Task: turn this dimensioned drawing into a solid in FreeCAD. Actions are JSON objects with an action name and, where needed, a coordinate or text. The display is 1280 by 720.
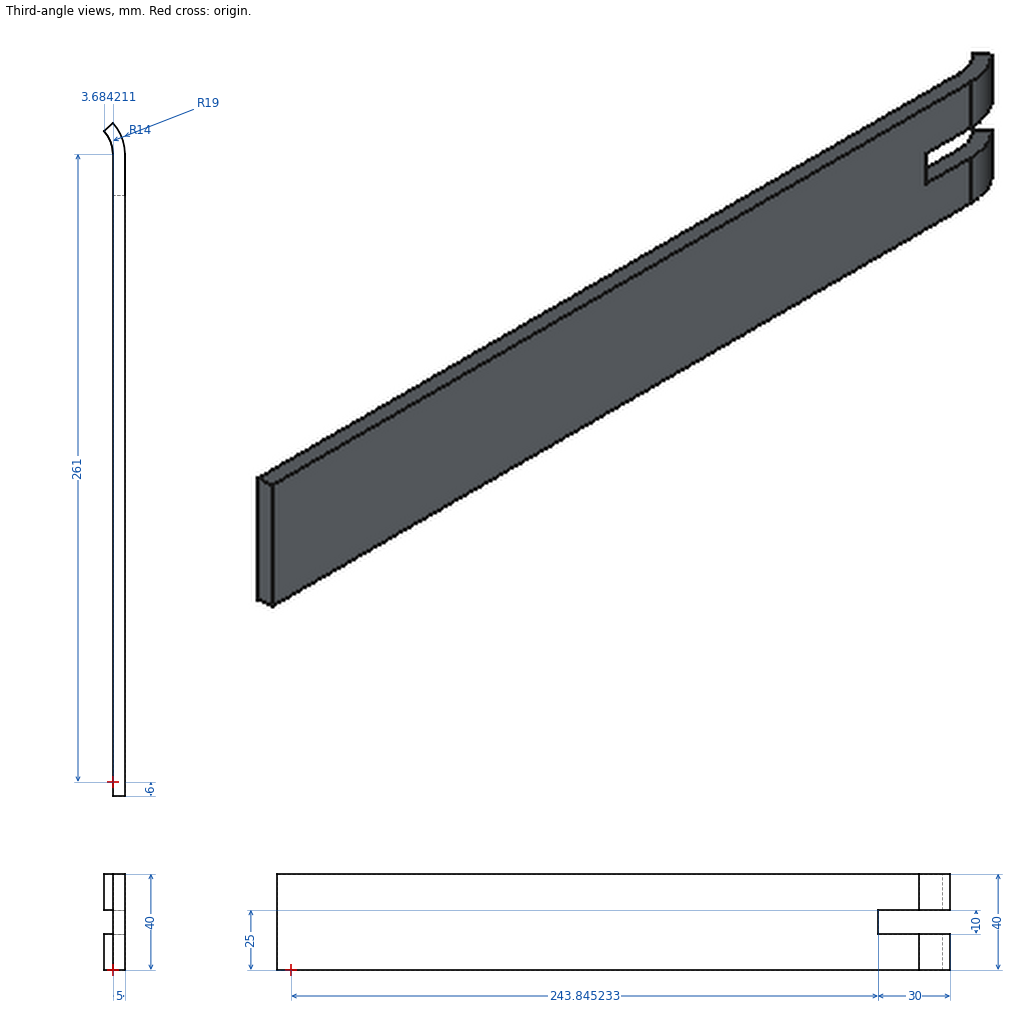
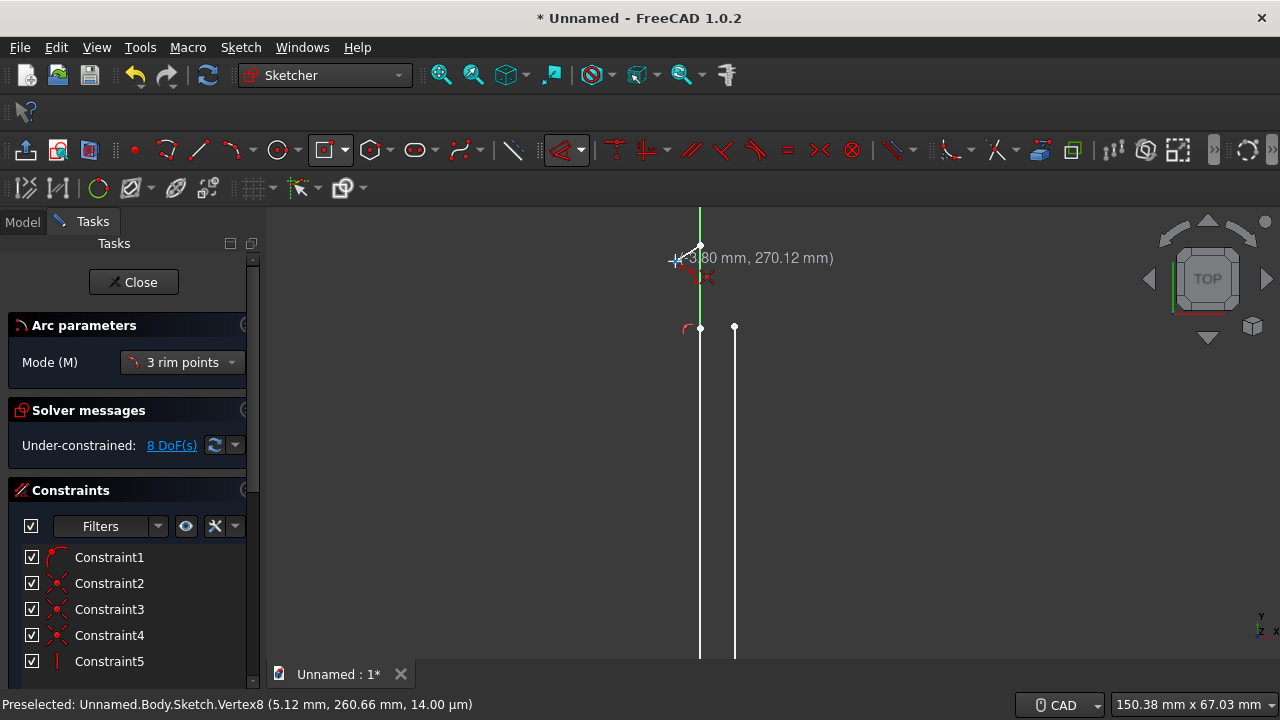
{"action": "left_click", "coordinate": [675, 262]}
{"action": "left_click", "coordinate": [700, 329]}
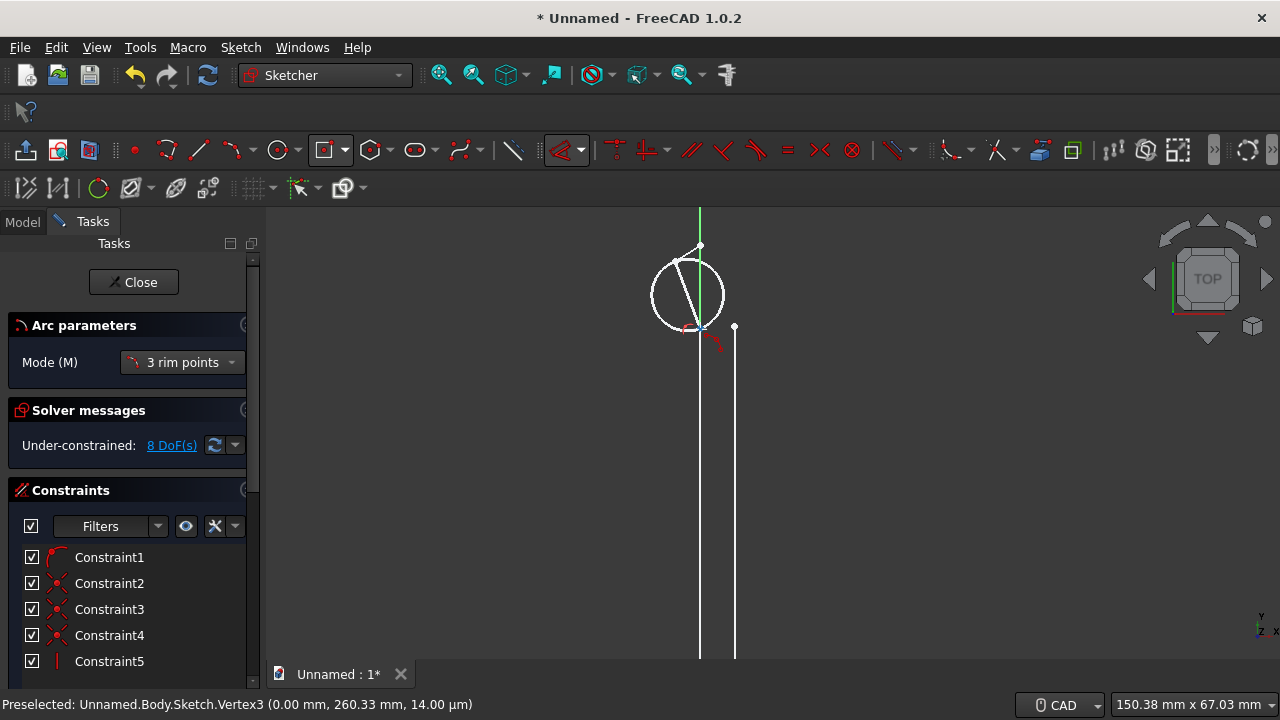
{"action": "scroll", "coordinate": [694, 290], "scroll_direction": "up", "scroll_amount": 5}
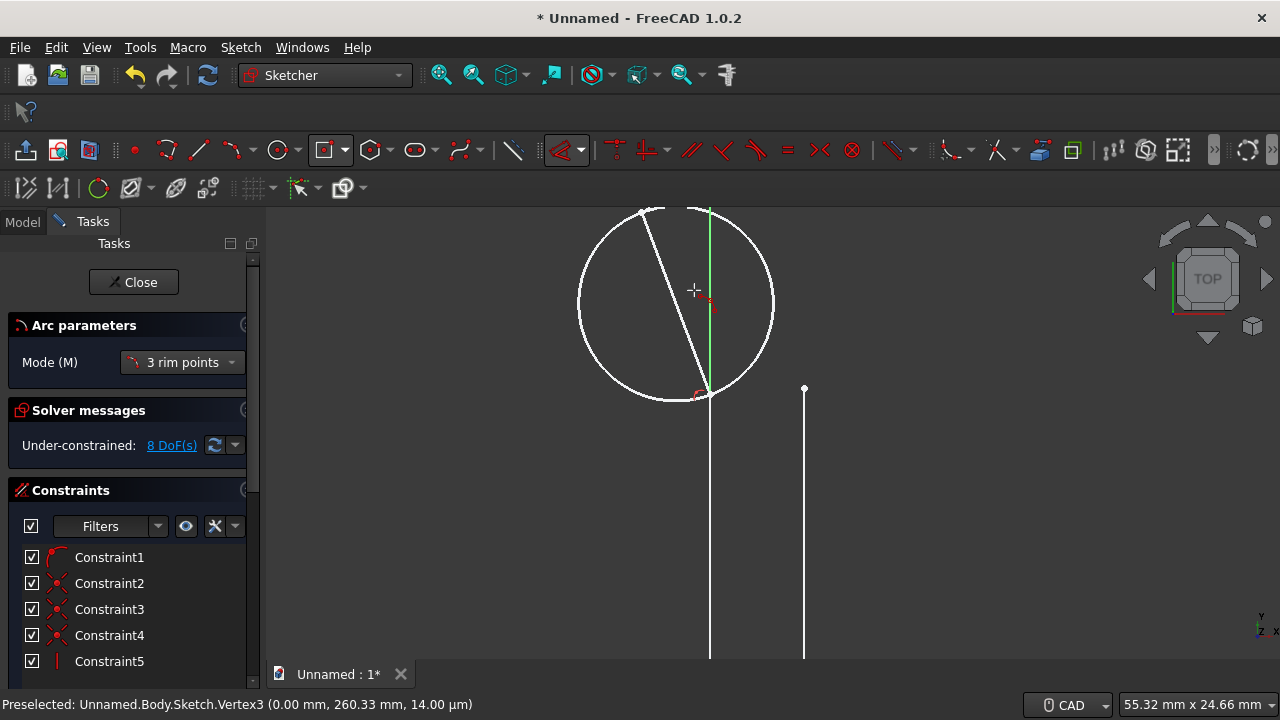
{"action": "left_click", "coordinate": [693, 290]}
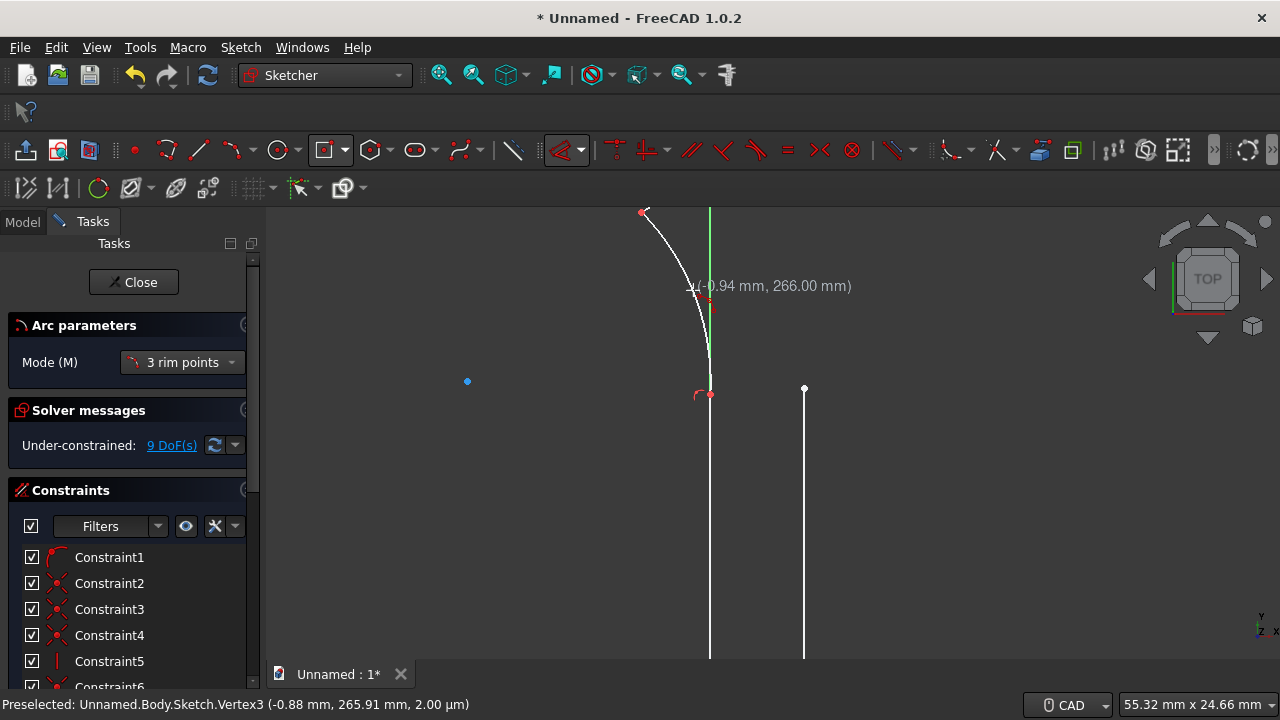
{"action": "scroll", "coordinate": [703, 289], "scroll_direction": "down", "scroll_amount": 14}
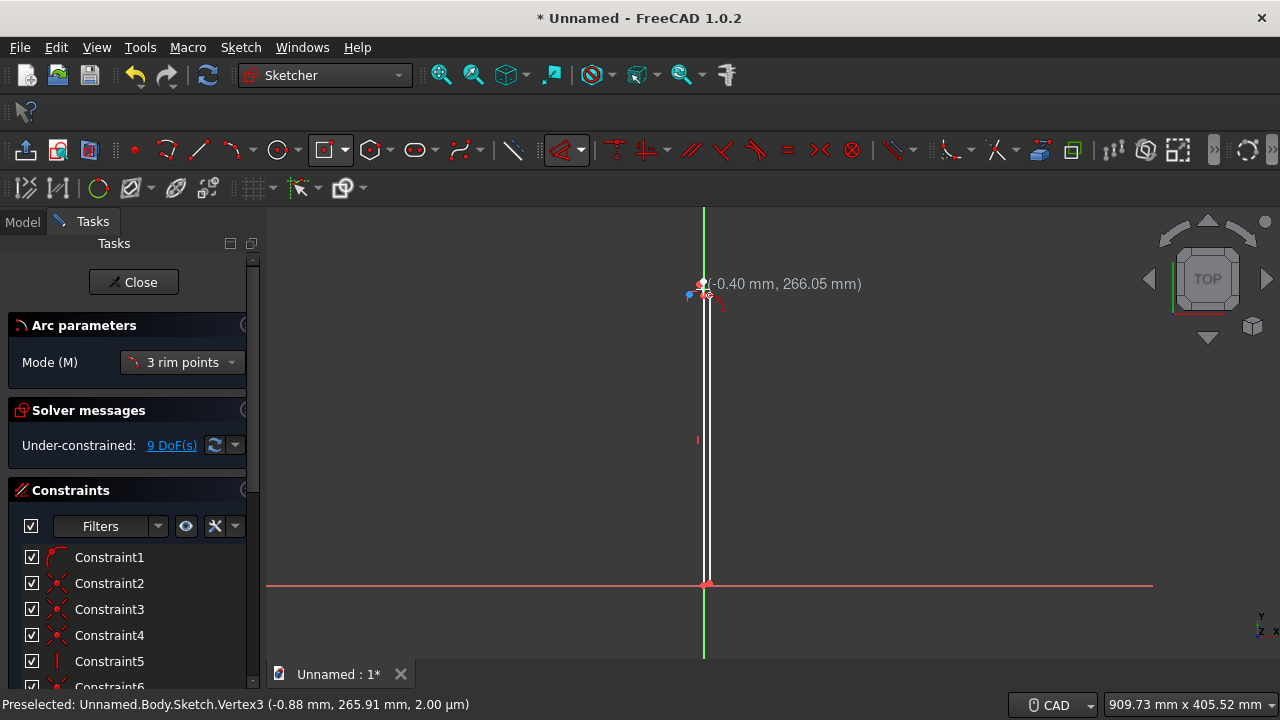
{"action": "scroll", "coordinate": [709, 295], "scroll_direction": "up", "scroll_amount": 6}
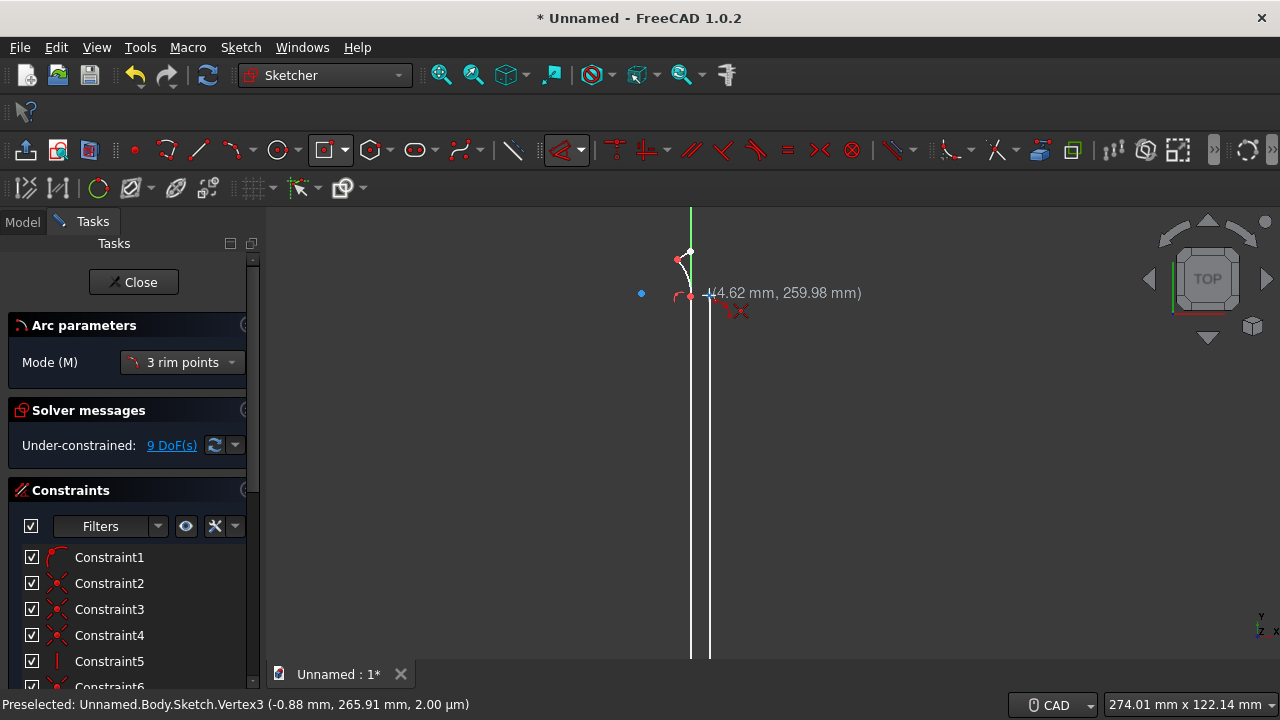
{"action": "left_click", "coordinate": [710, 295]}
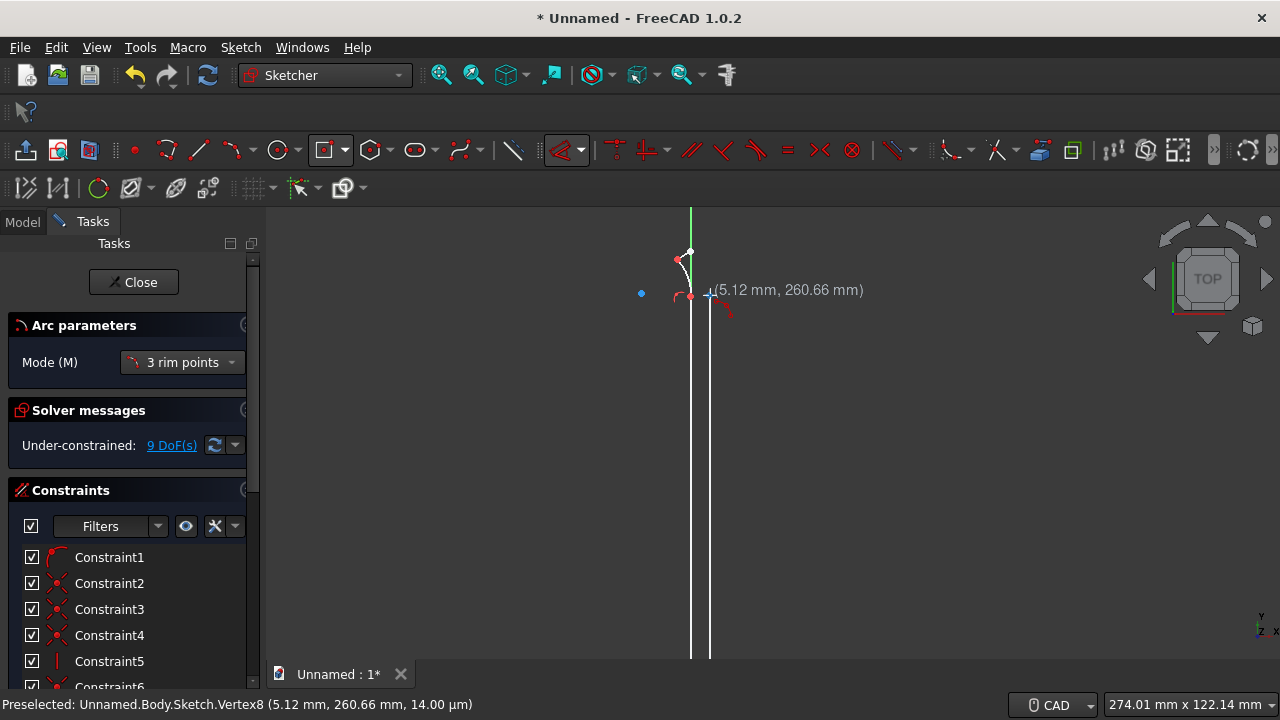
{"action": "scroll", "coordinate": [691, 247], "scroll_direction": "up", "scroll_amount": 3}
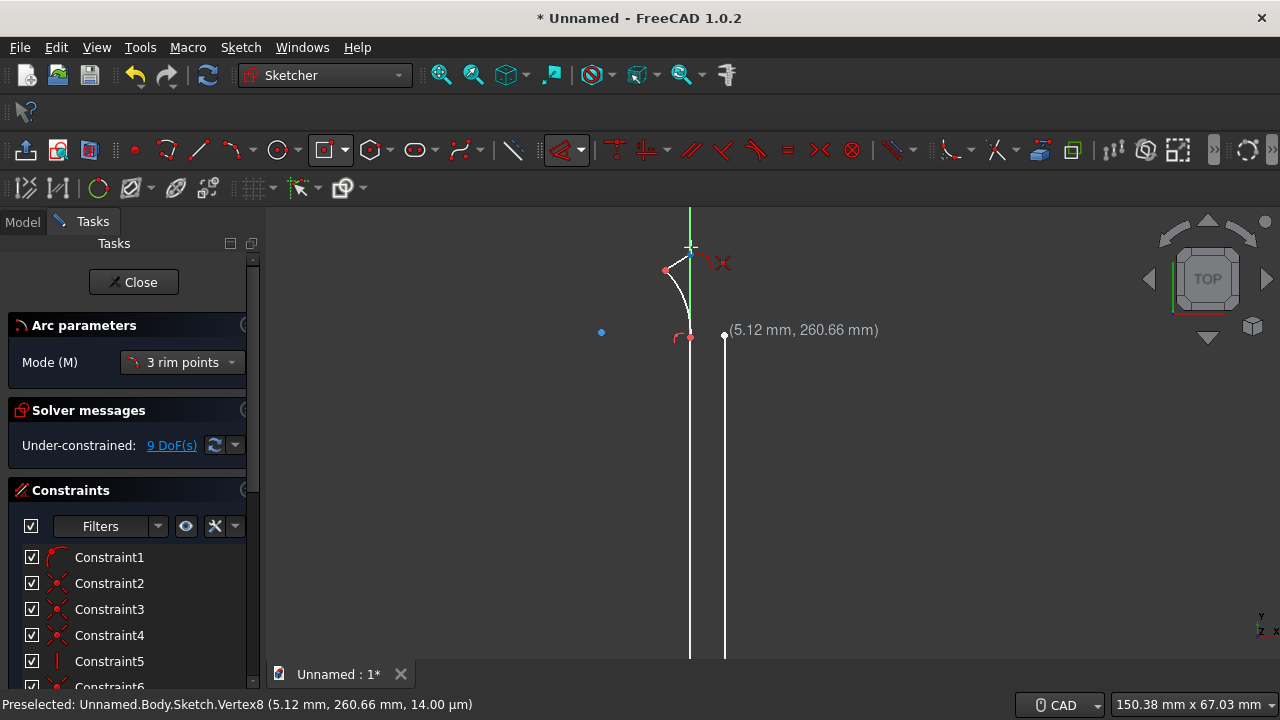
{"action": "left_click", "coordinate": [690, 254]}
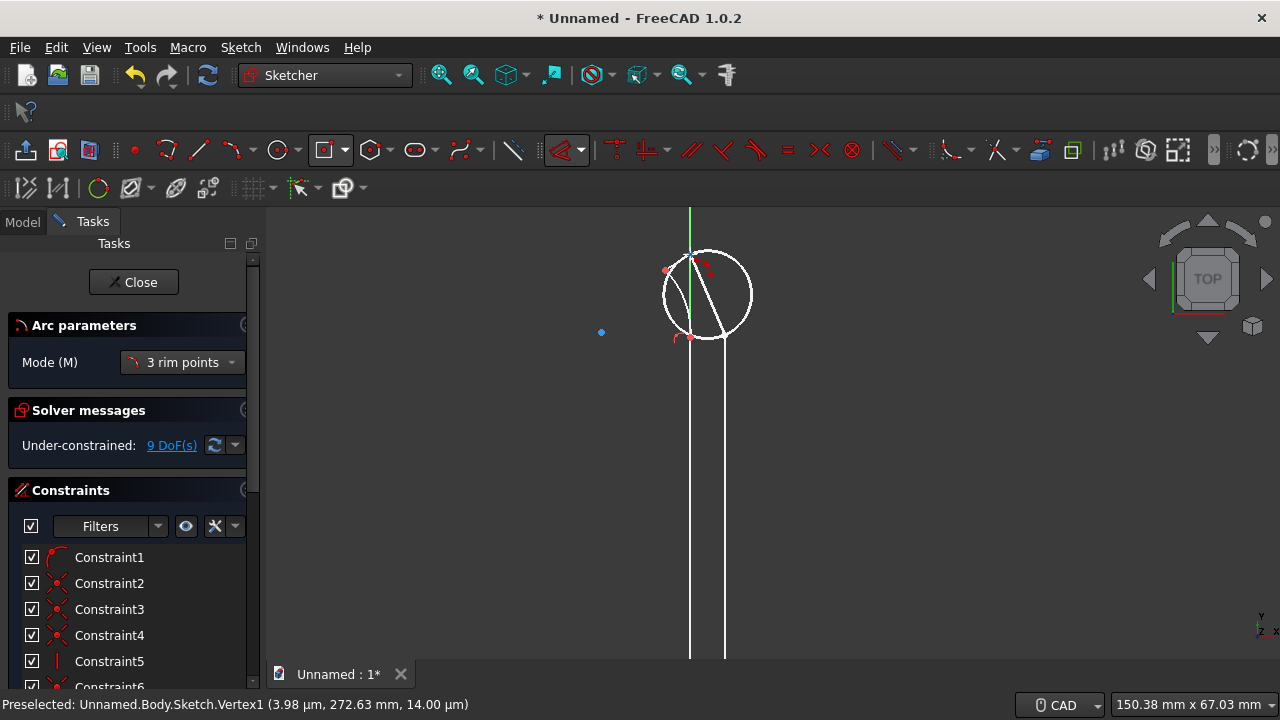
{"action": "scroll", "coordinate": [715, 286], "scroll_direction": "up", "scroll_amount": 3}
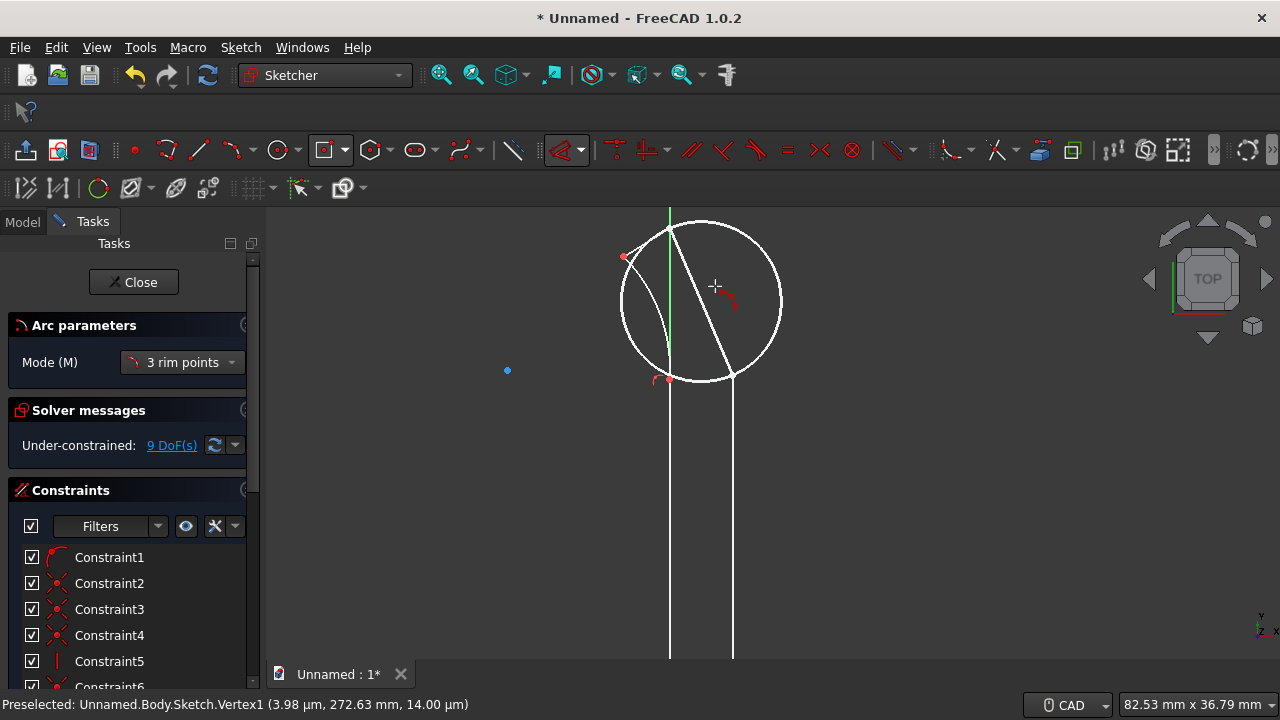
{"action": "left_click", "coordinate": [715, 286]}
{"action": "key", "text": "Escape"}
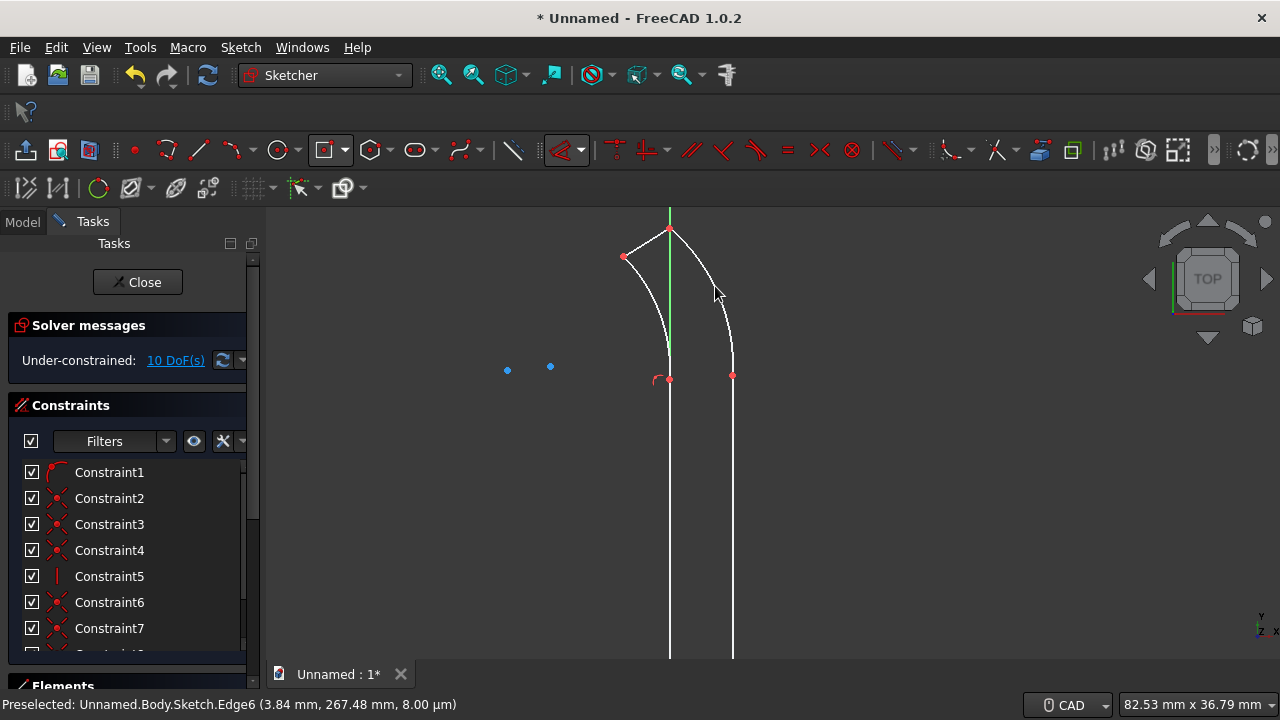
{"action": "scroll", "coordinate": [707, 287], "scroll_direction": "down", "scroll_amount": 12}